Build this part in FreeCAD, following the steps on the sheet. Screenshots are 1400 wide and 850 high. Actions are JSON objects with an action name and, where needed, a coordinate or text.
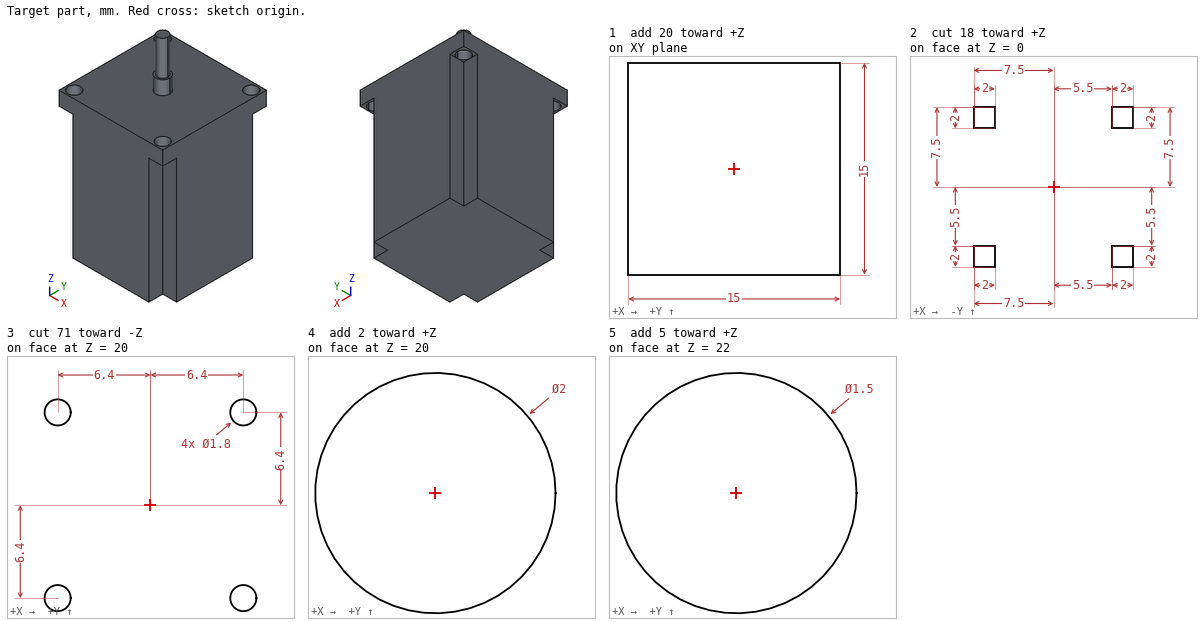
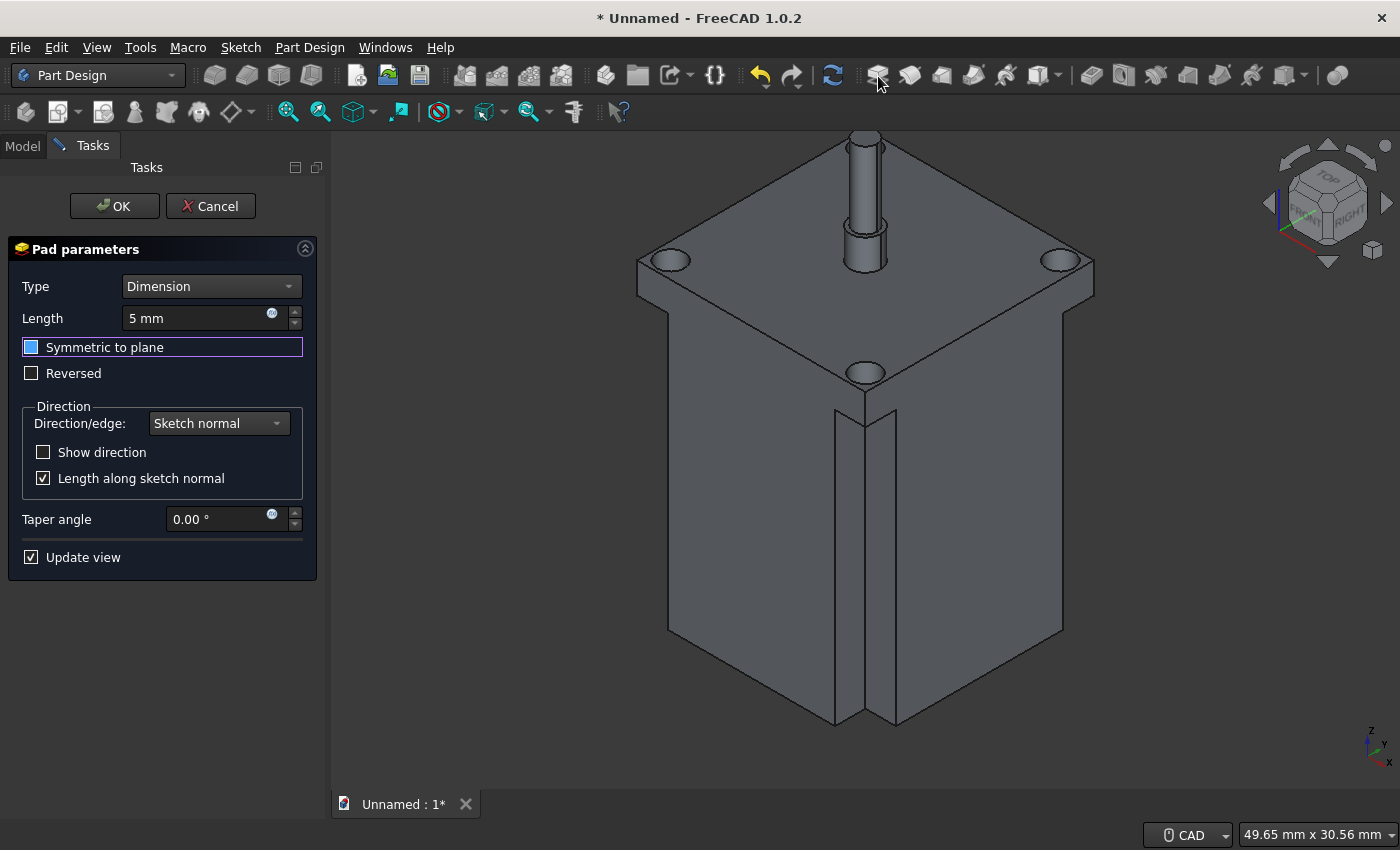
{"action": "left_click", "coordinate": [115, 206]}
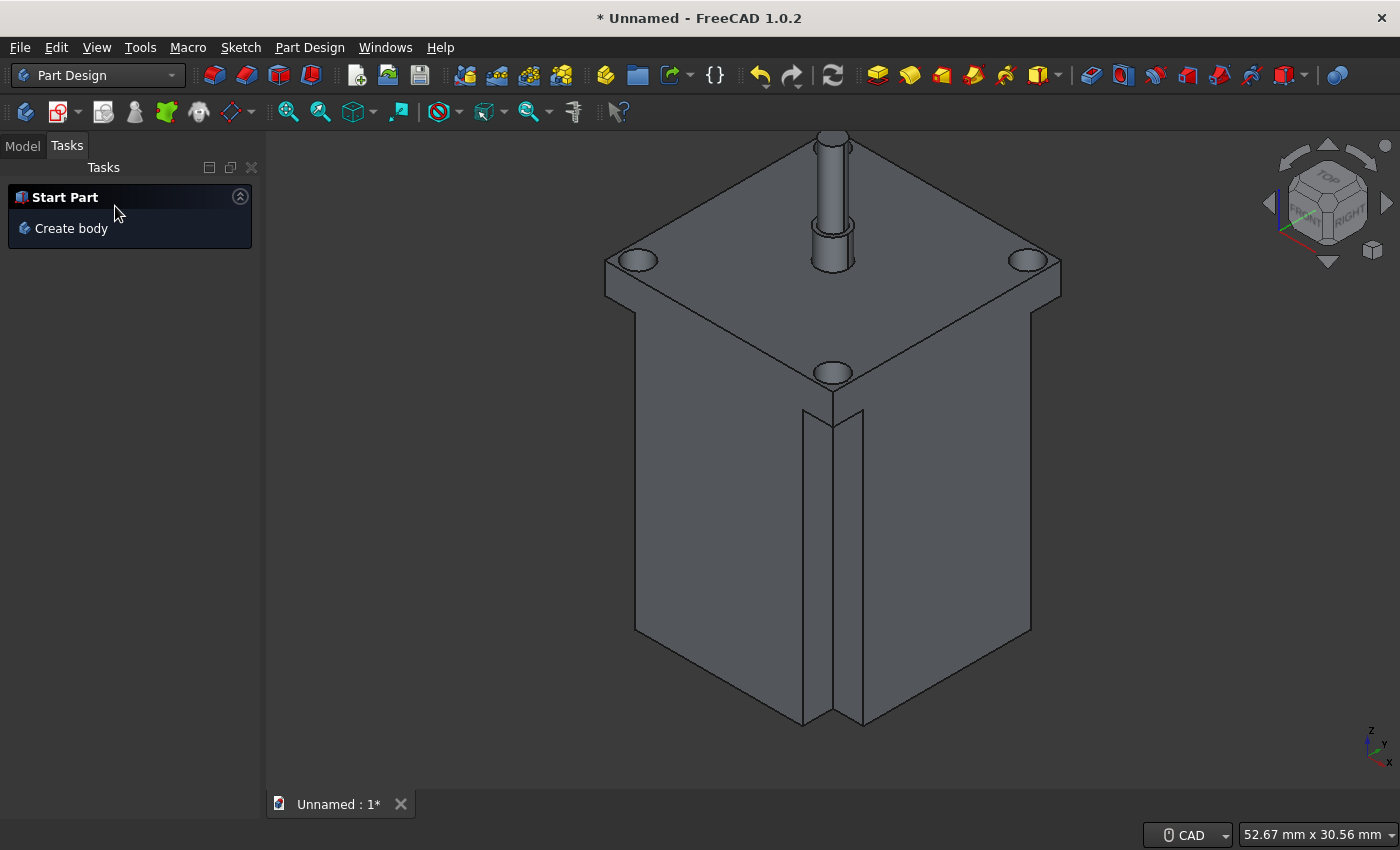
{"action": "key", "text": "v f"}